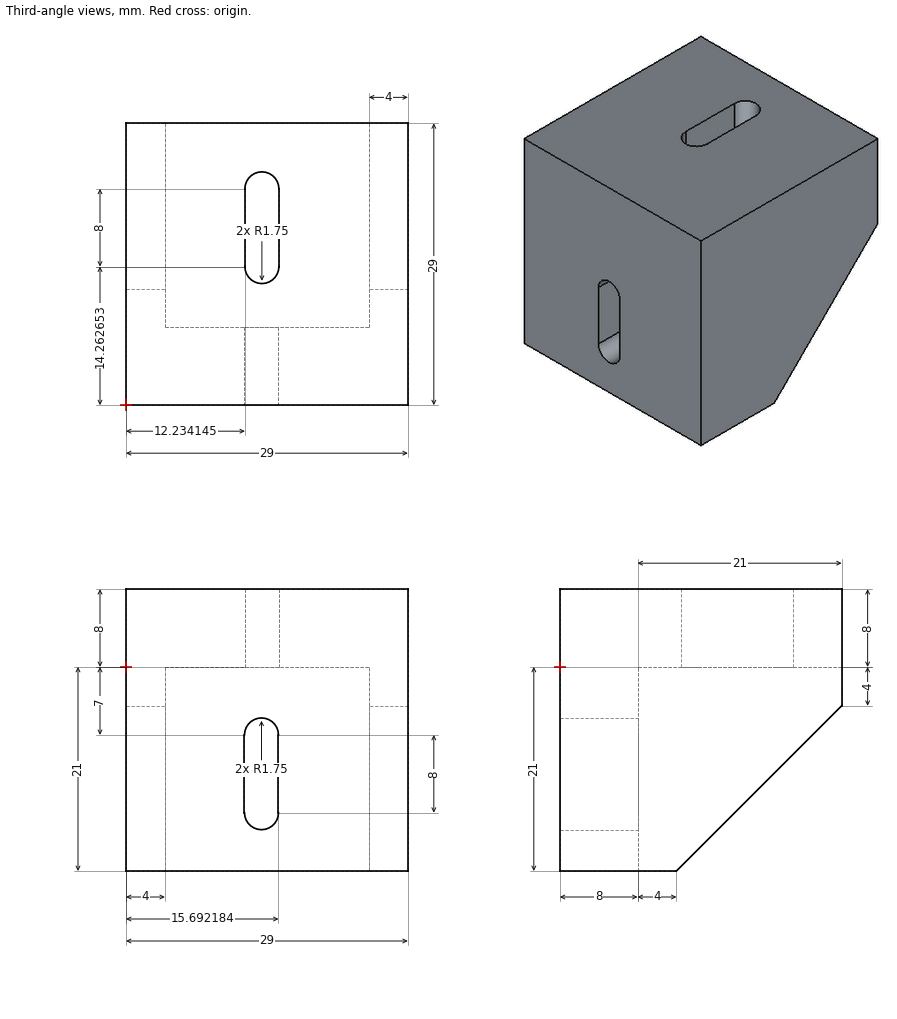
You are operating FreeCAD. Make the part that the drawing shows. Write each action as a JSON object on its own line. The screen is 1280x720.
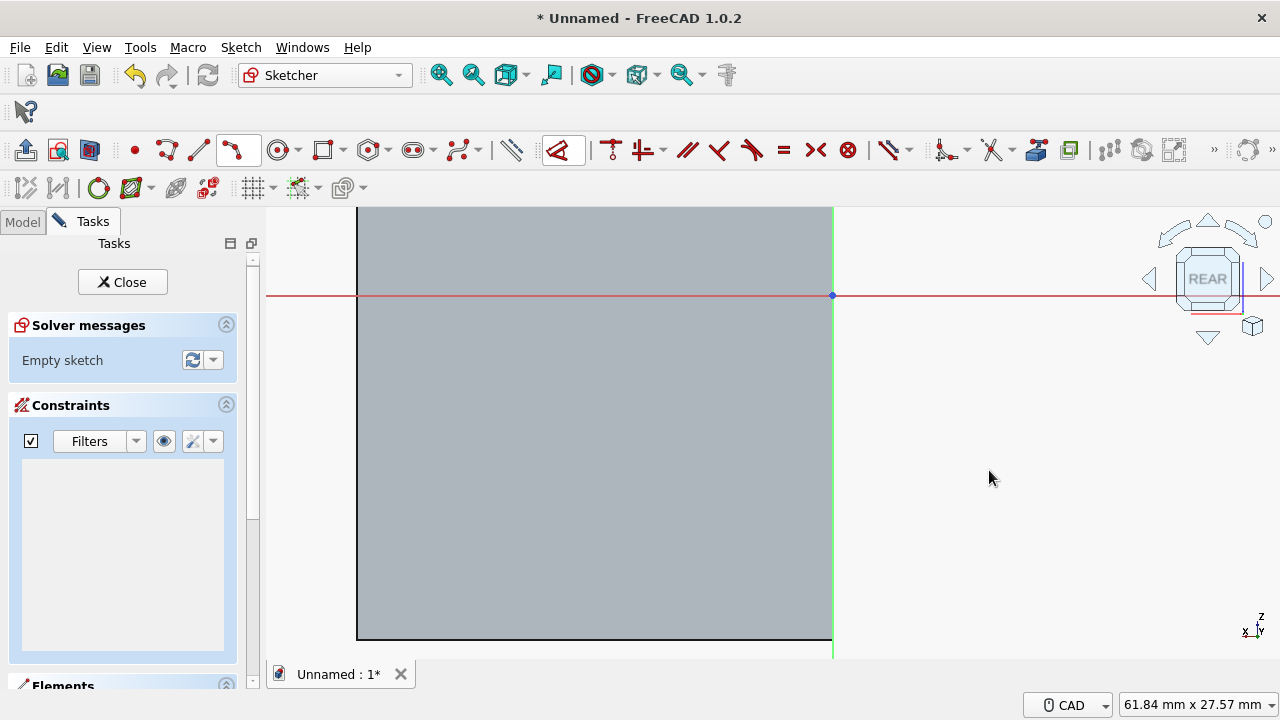
{"action": "left_click", "coordinate": [414, 150]}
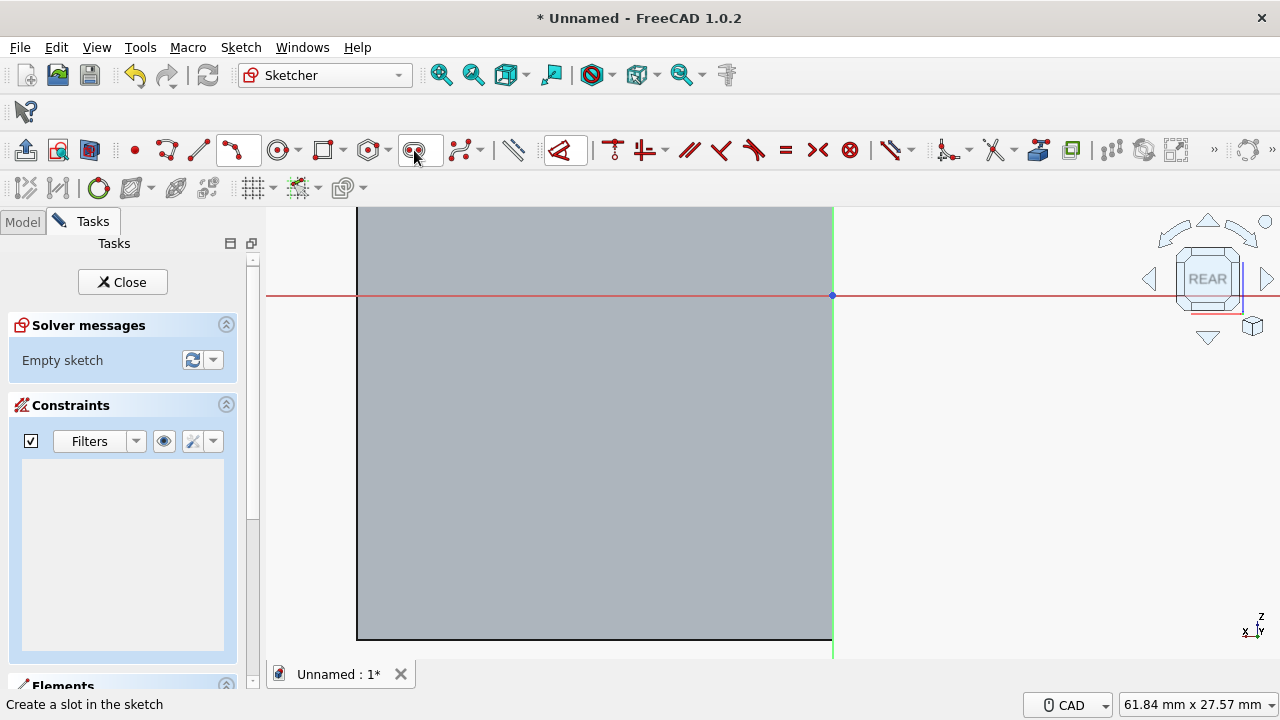
{"action": "left_click", "coordinate": [604, 541]}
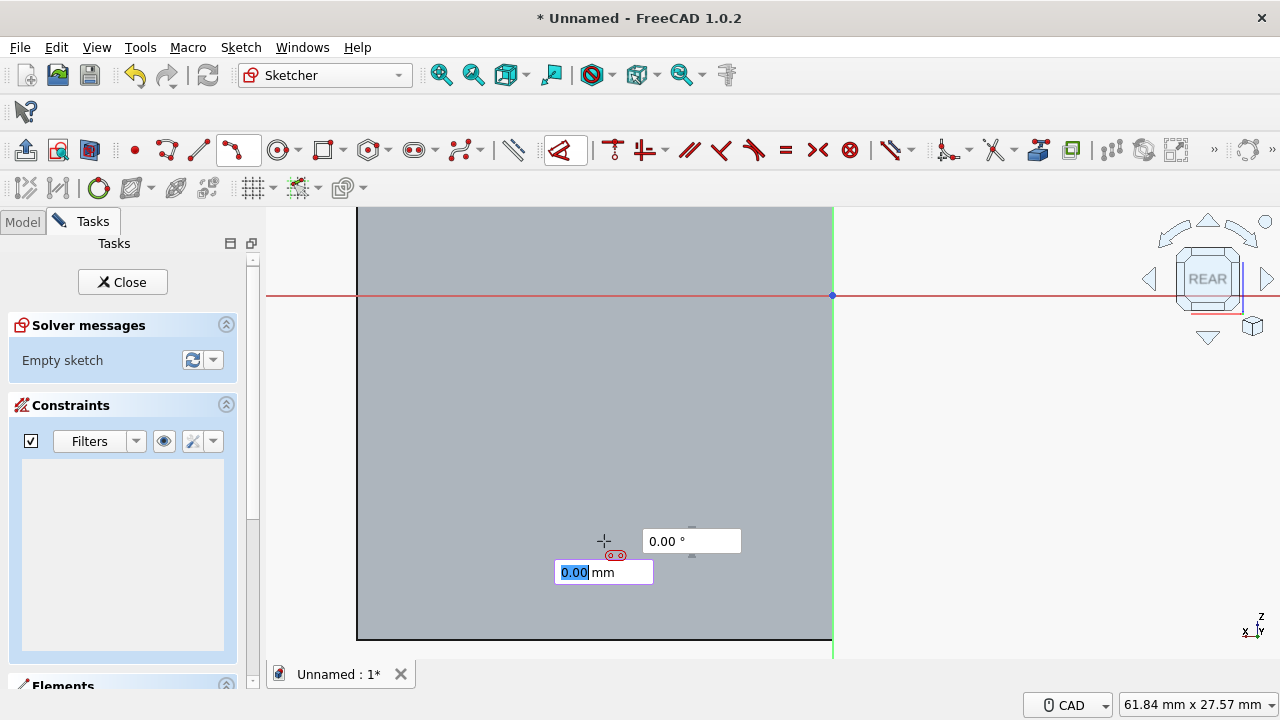
{"action": "left_click", "coordinate": [604, 410]}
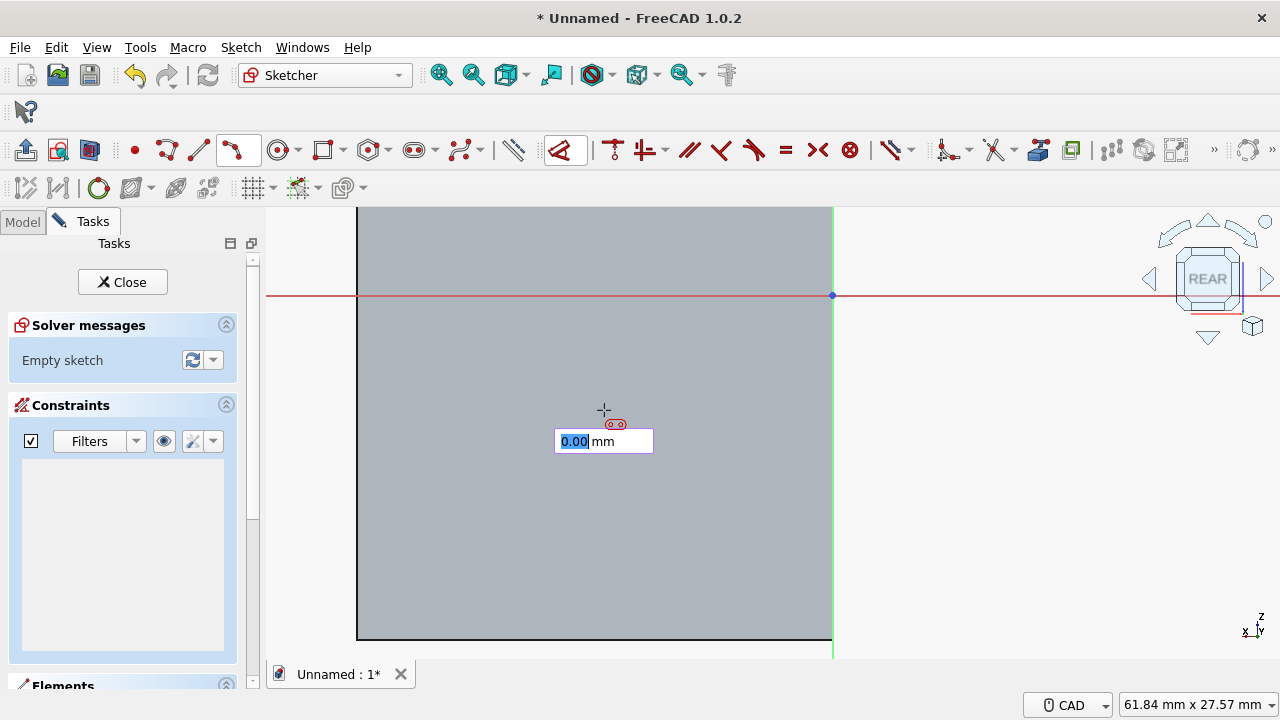
{"action": "left_click", "coordinate": [633, 476]}
{"action": "key", "text": "Escape"}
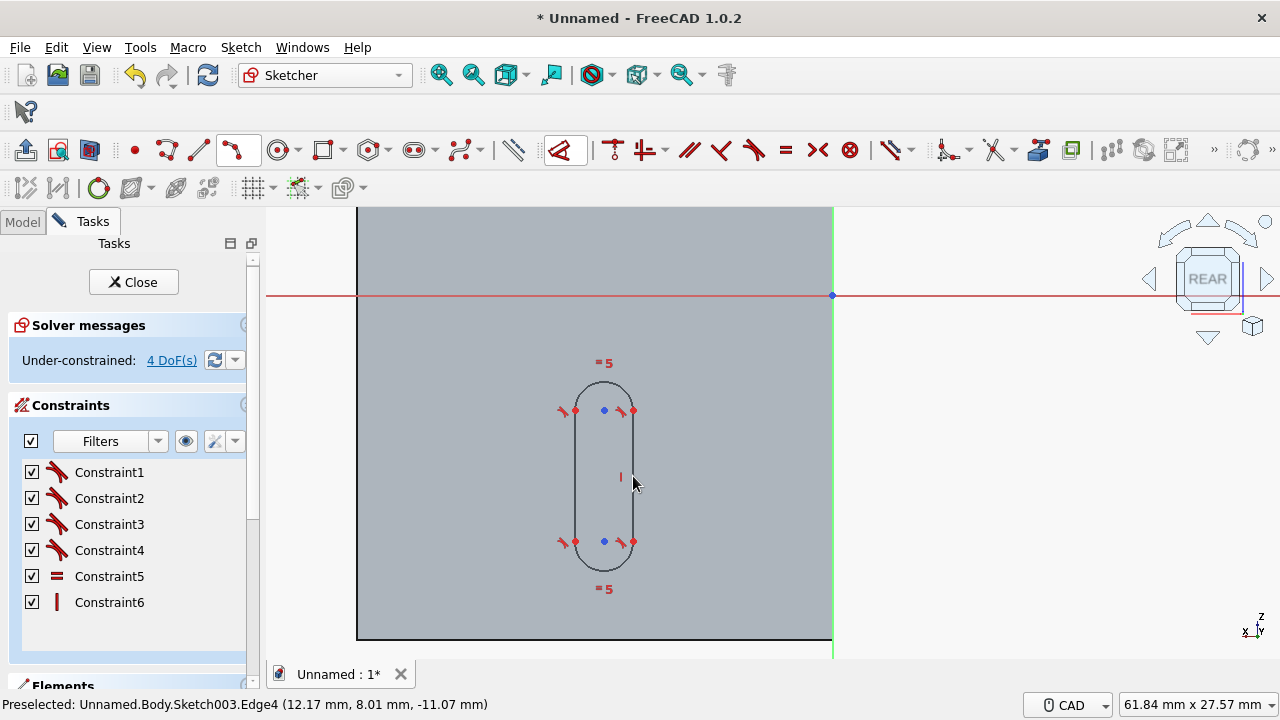
{"action": "scroll", "coordinate": [587, 565], "scroll_direction": "up", "scroll_amount": 2}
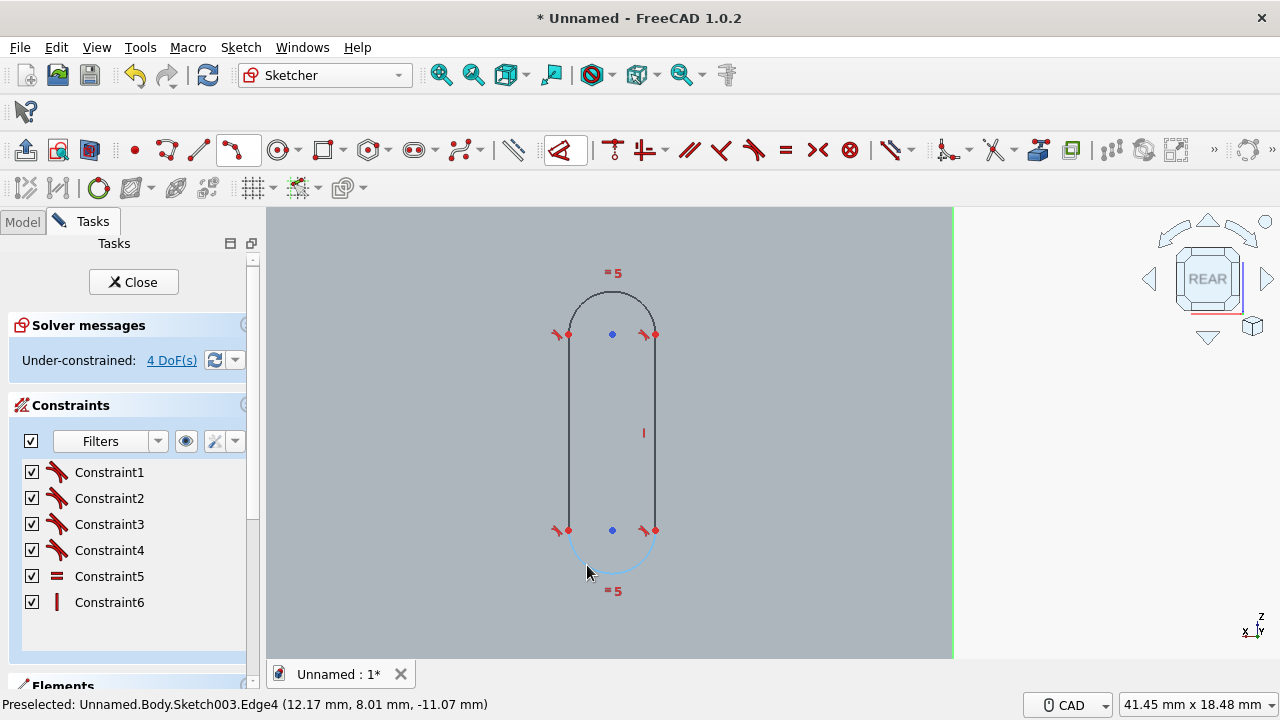
{"action": "left_click", "coordinate": [587, 565]}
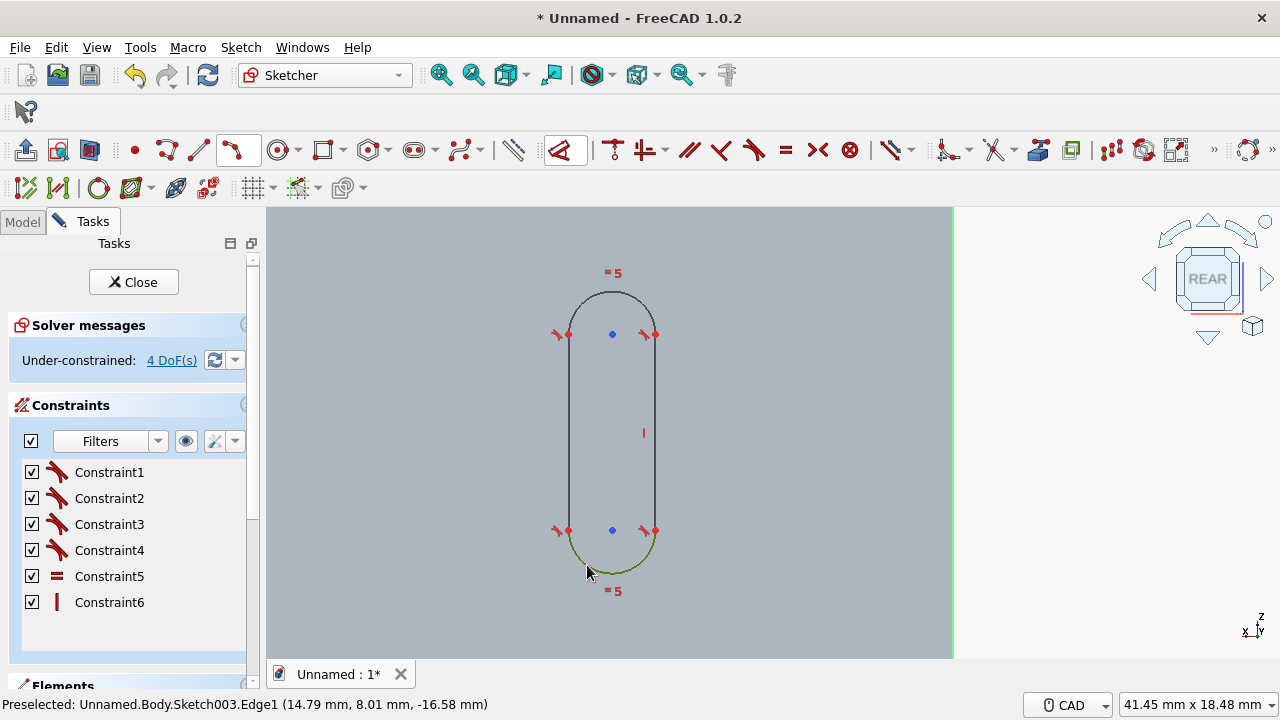
{"action": "left_click", "coordinate": [582, 150]}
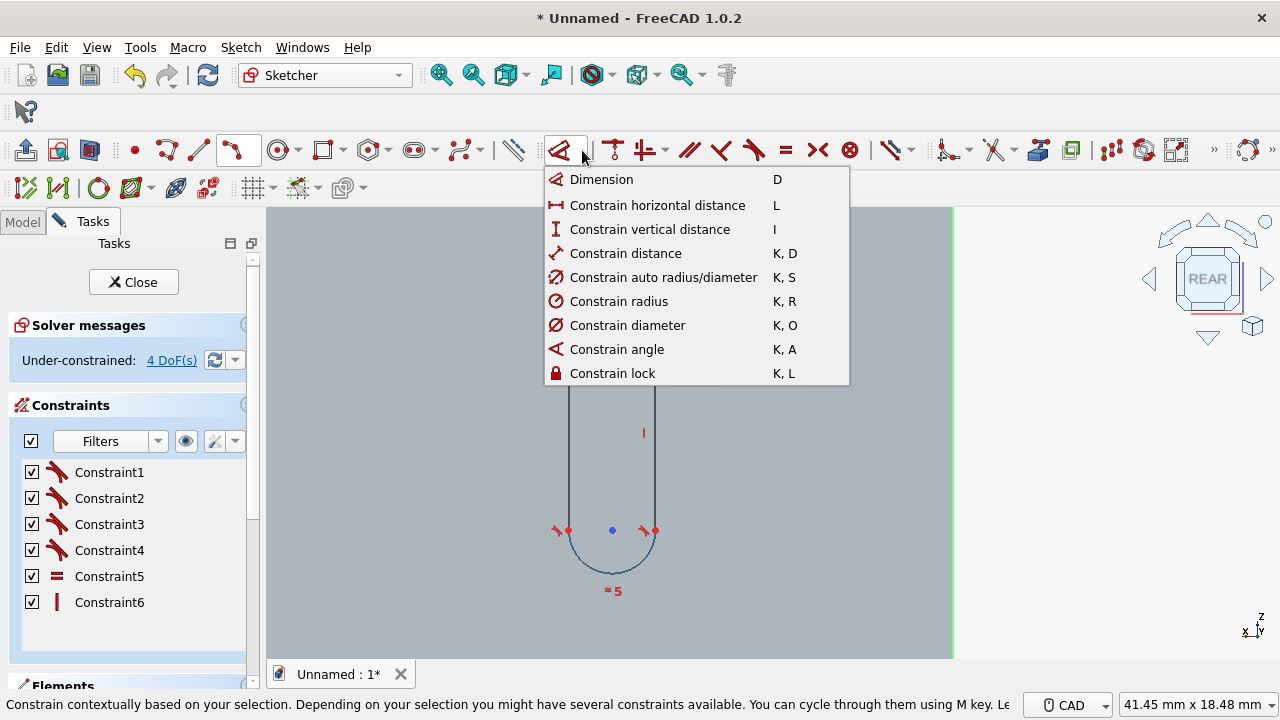
{"action": "left_click", "coordinate": [697, 301]}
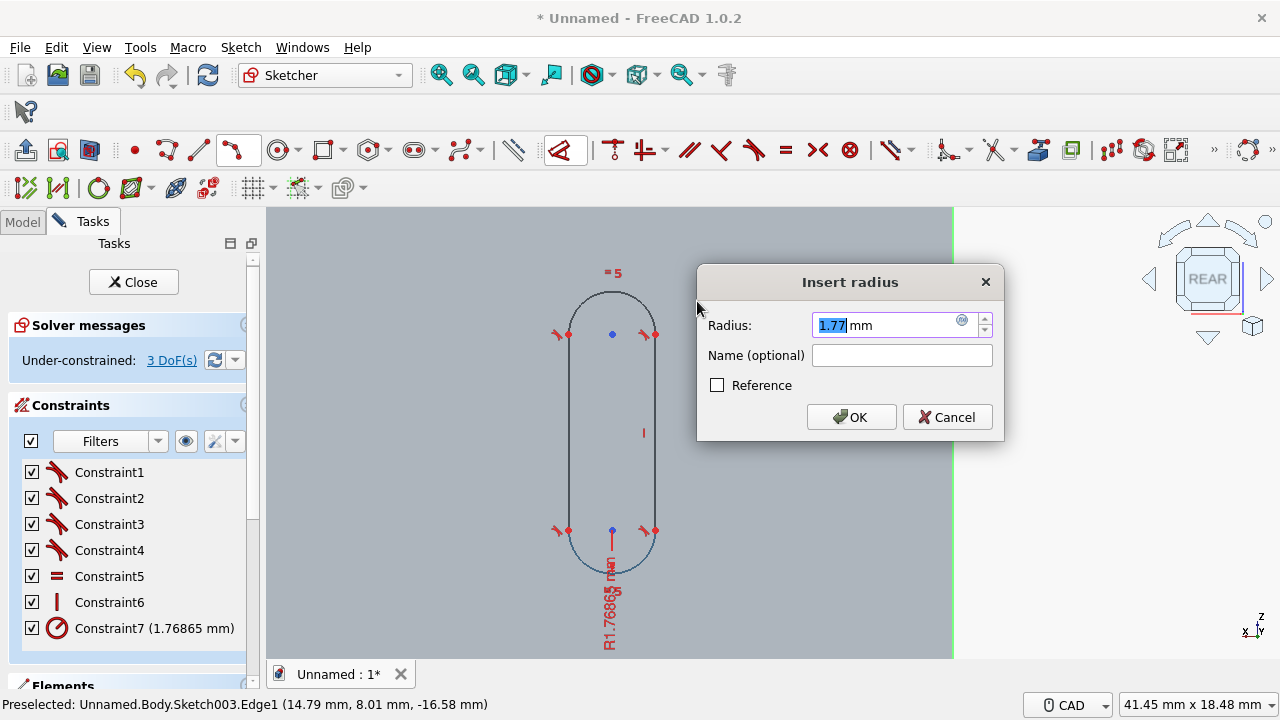
{"action": "type", "text": "1.75"}
{"action": "key", "text": "Return"}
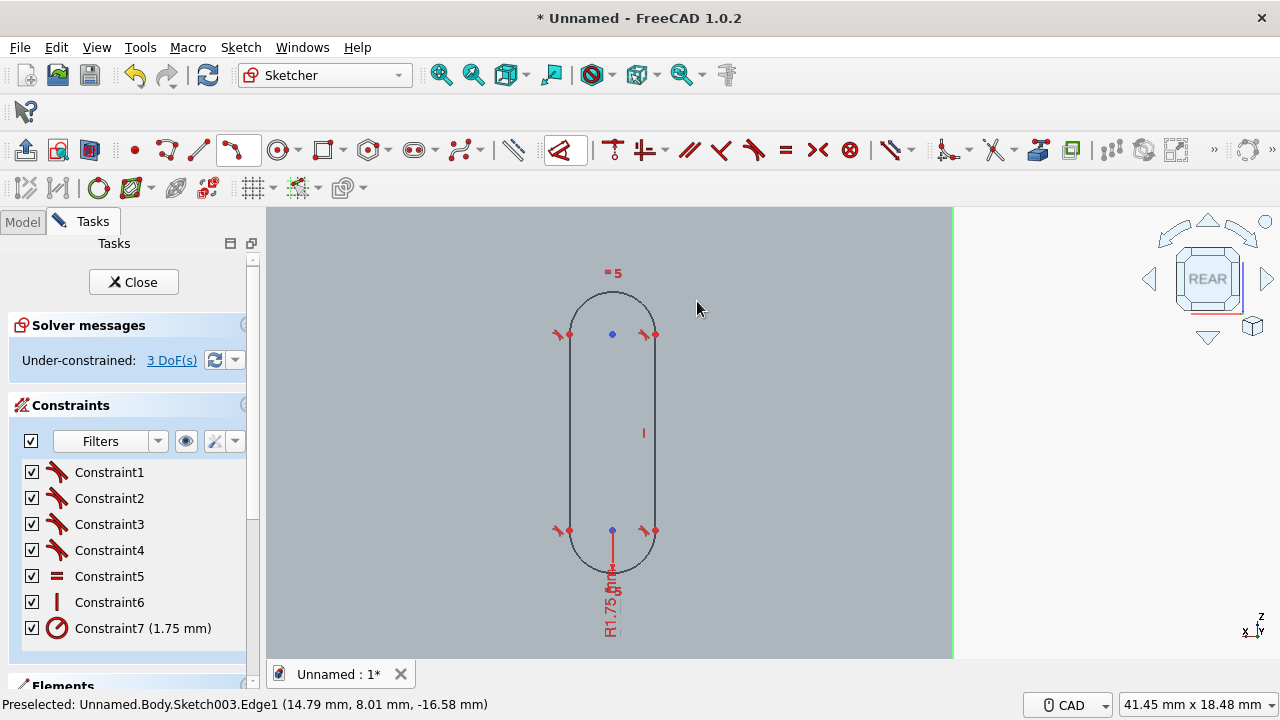
{"action": "left_click", "coordinate": [570, 472]}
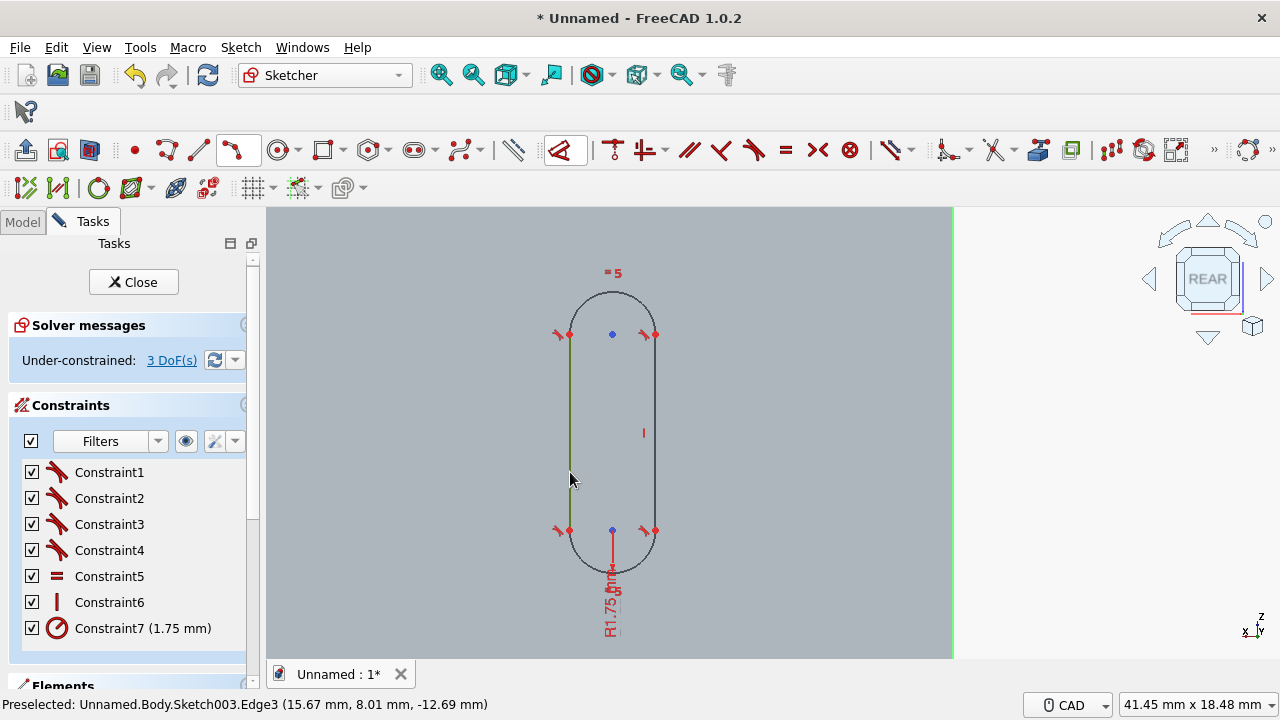
{"action": "key", "text": "i"}